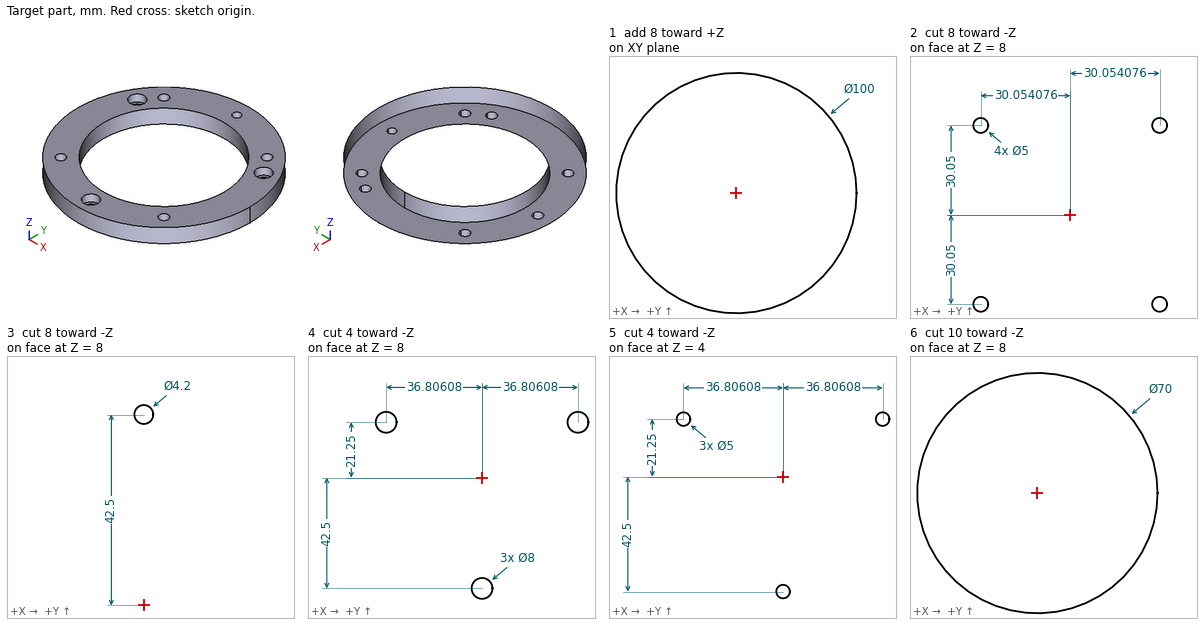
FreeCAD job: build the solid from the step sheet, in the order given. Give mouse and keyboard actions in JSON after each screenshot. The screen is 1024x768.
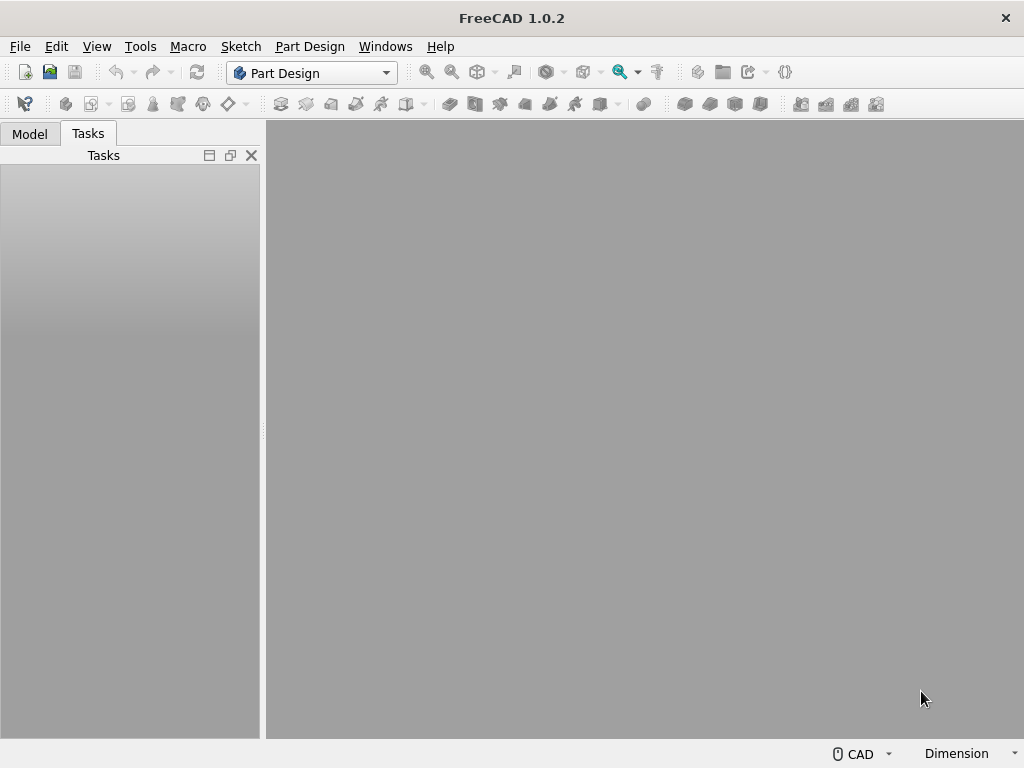
{"action": "left_click", "coordinate": [25, 72]}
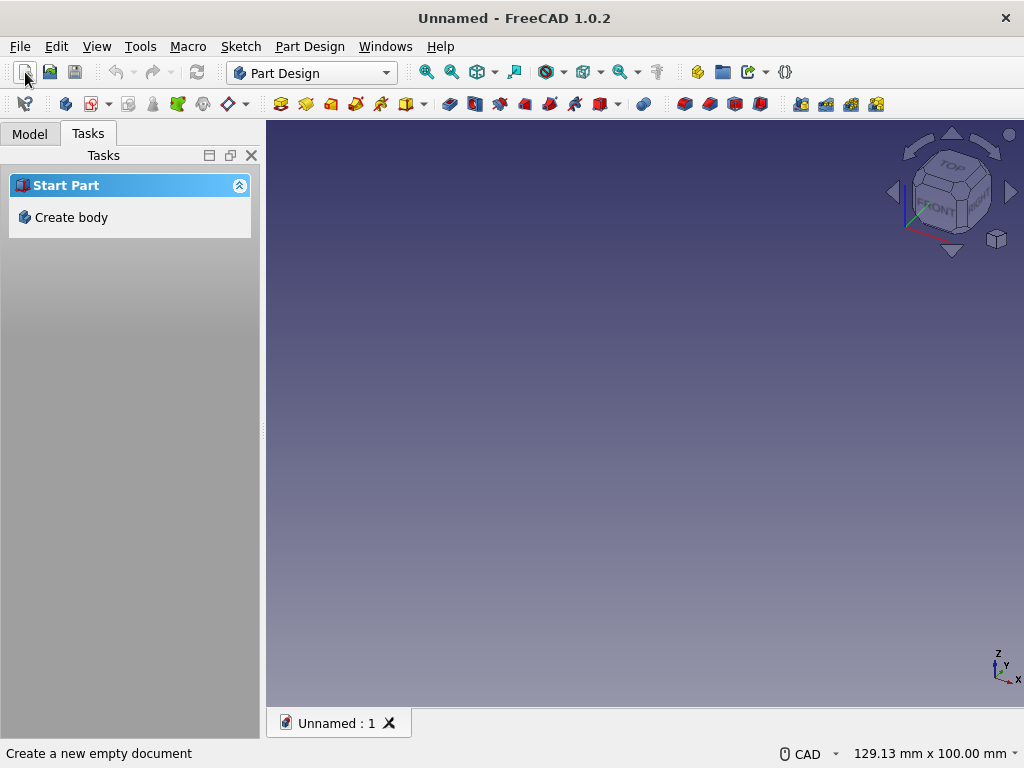
{"action": "left_click", "coordinate": [90, 104]}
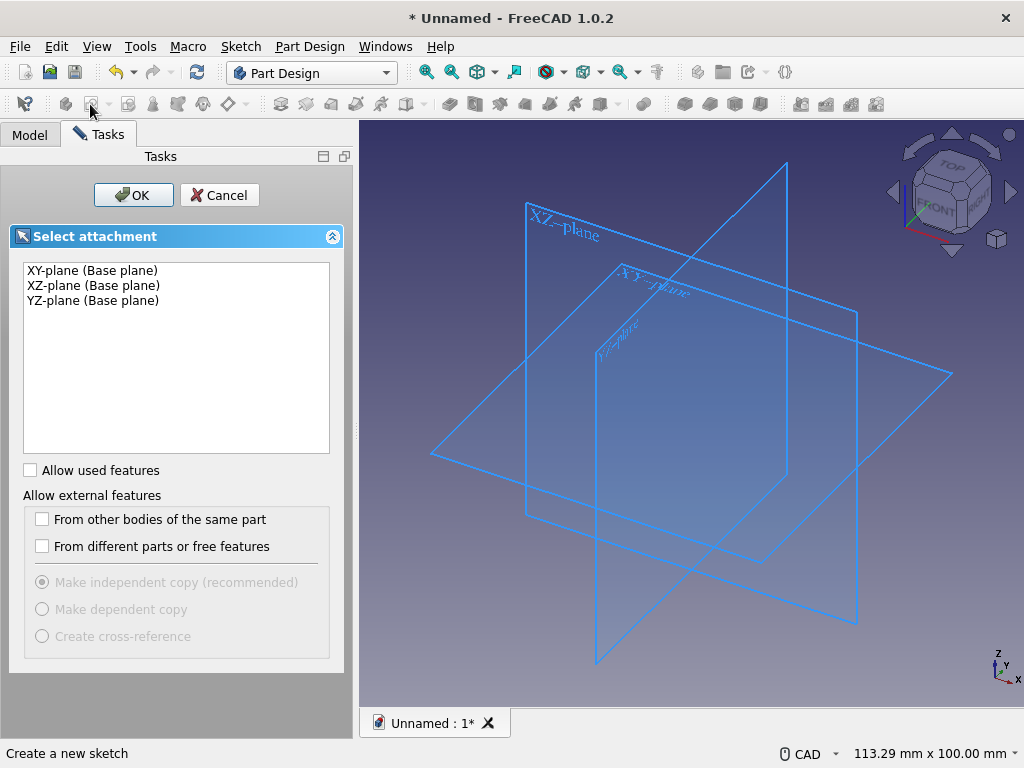
{"action": "left_click", "coordinate": [84, 270]}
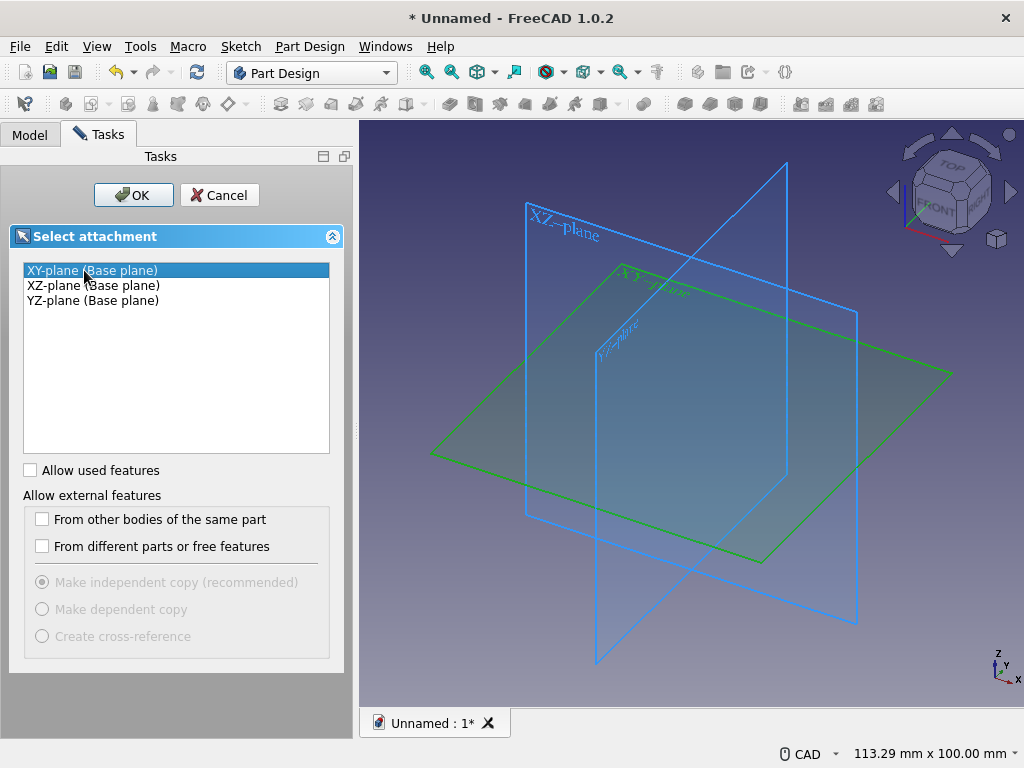
{"action": "left_click", "coordinate": [134, 195]}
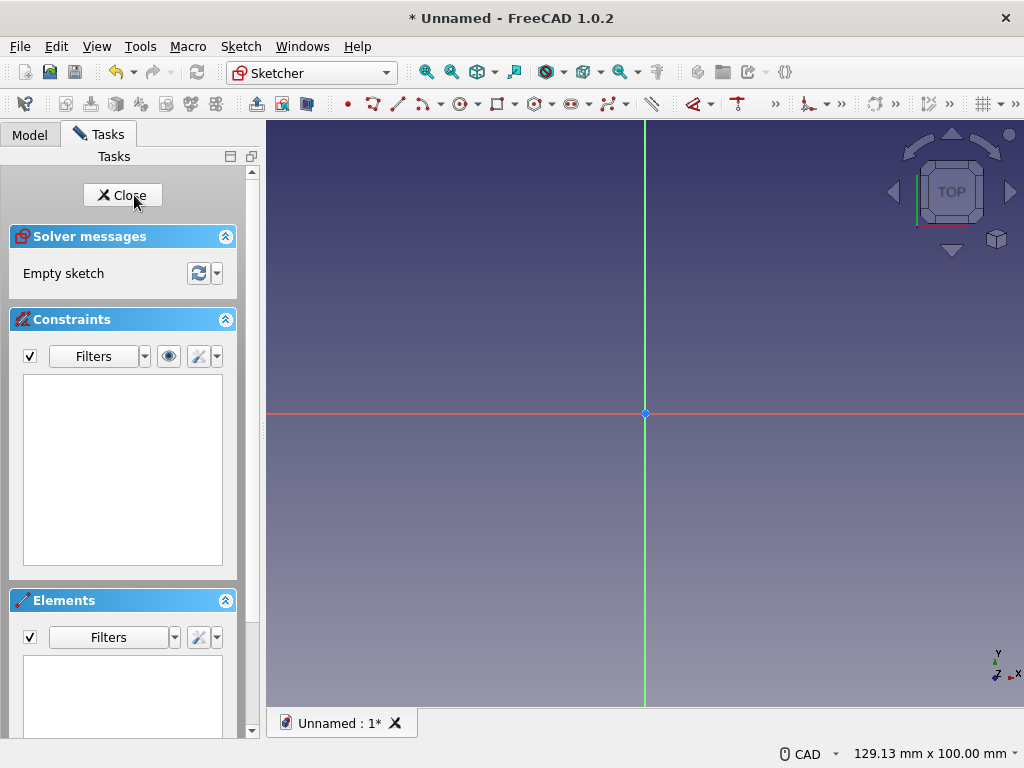
{"action": "scroll", "coordinate": [437, 414], "scroll_direction": "down", "scroll_amount": 2}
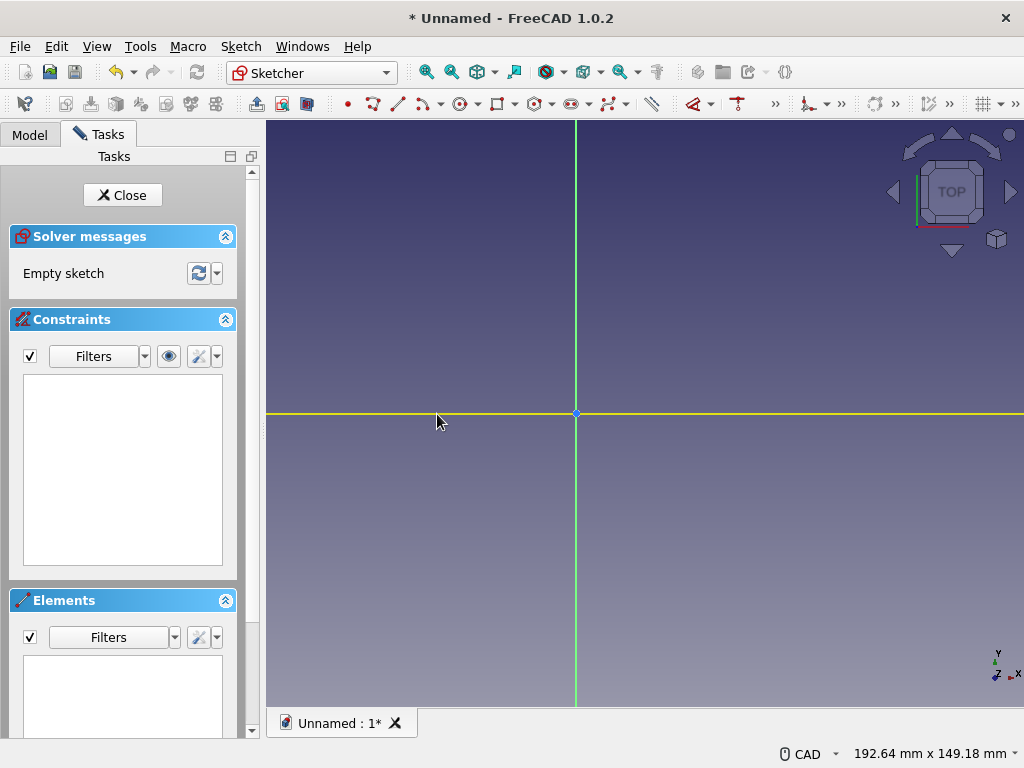
{"action": "key", "text": "g c"}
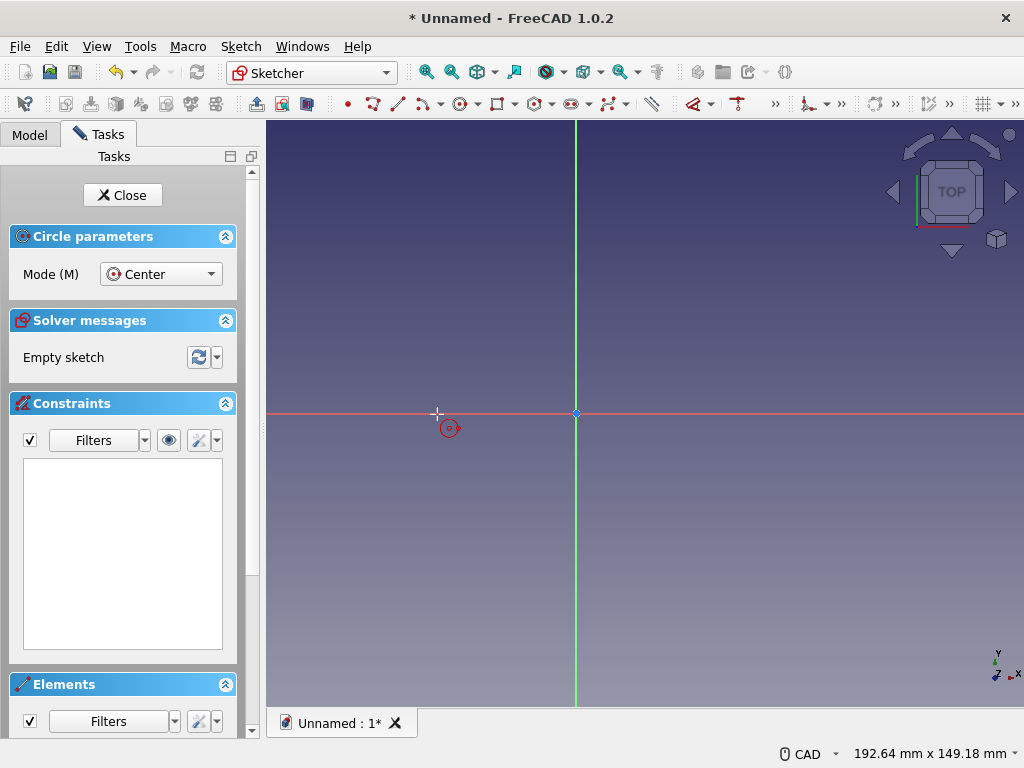
{"action": "left_click", "coordinate": [577, 414]}
{"action": "mouse_move", "coordinate": [716, 275]}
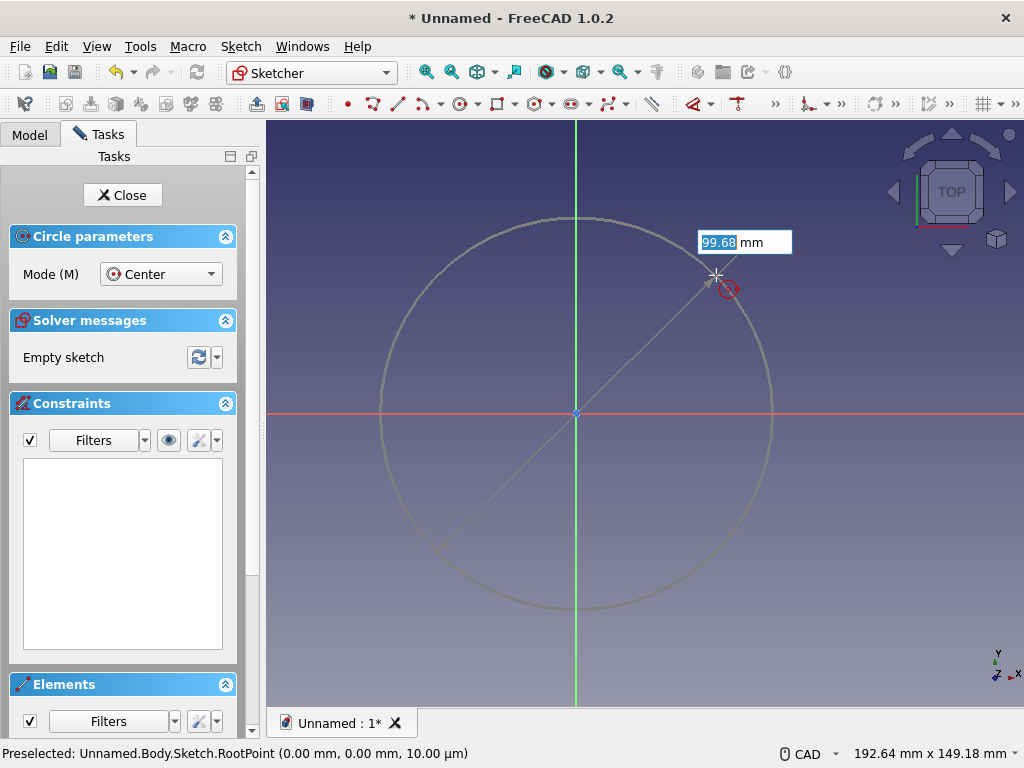
{"action": "type", "text": "100"}
{"action": "key", "text": "Return"}
{"action": "key", "text": "Escape"}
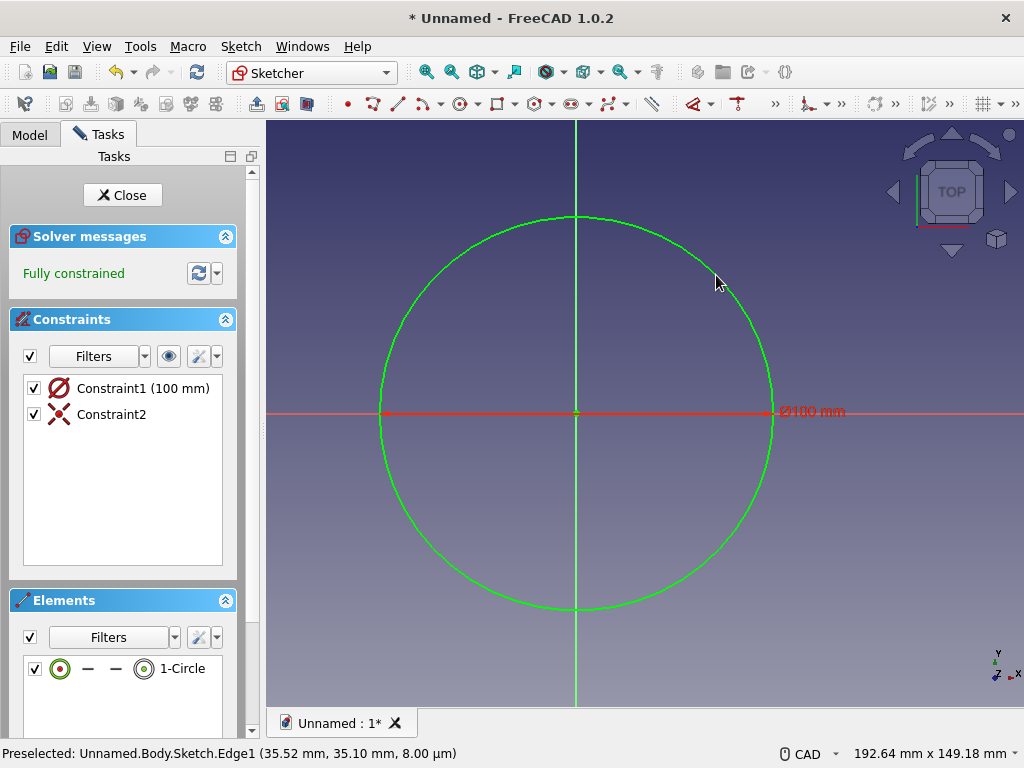
{"action": "left_click", "coordinate": [123, 195]}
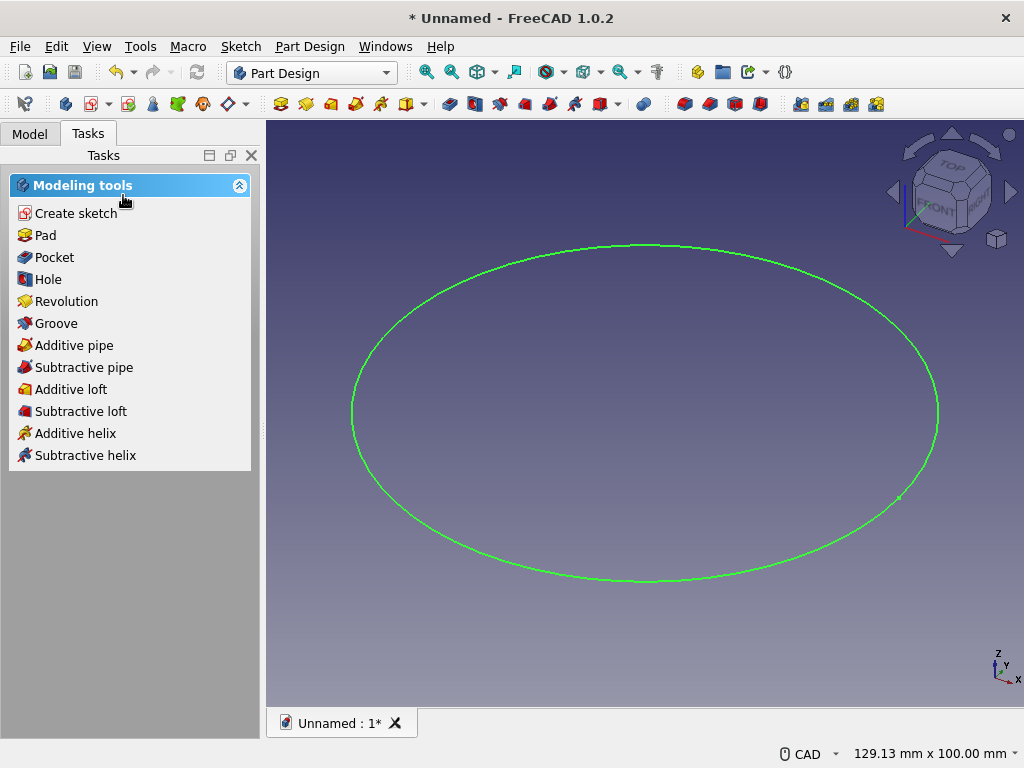
{"action": "left_click", "coordinate": [281, 104]}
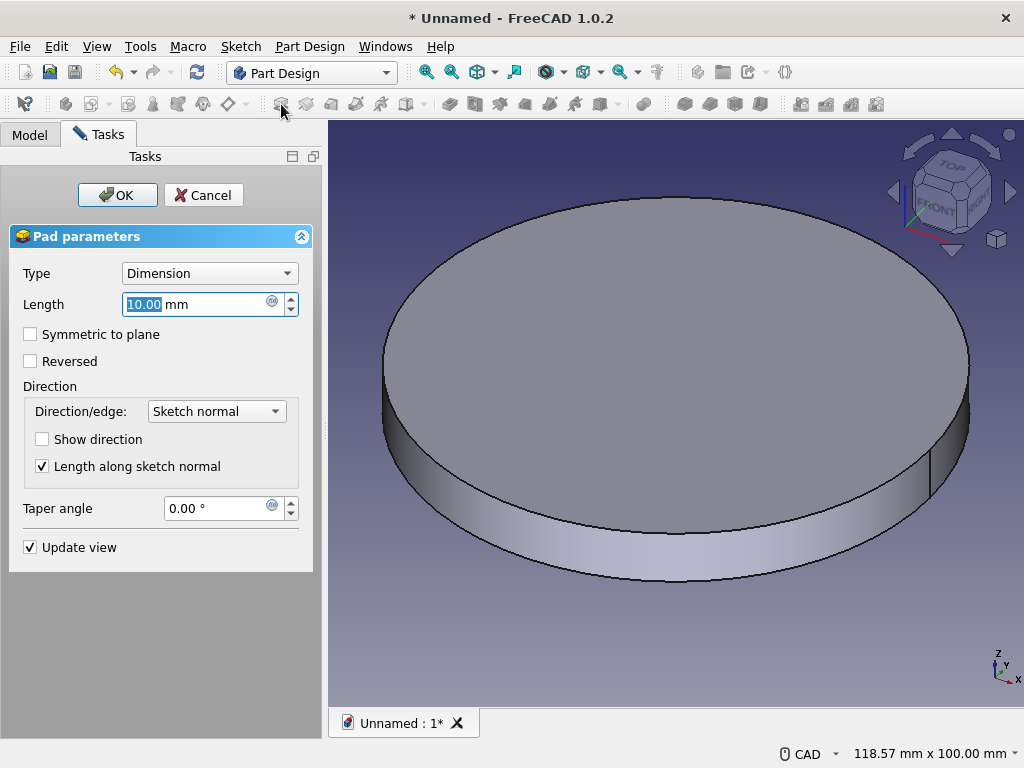
{"action": "type", "text": "8"}
{"action": "key", "text": "Tab"}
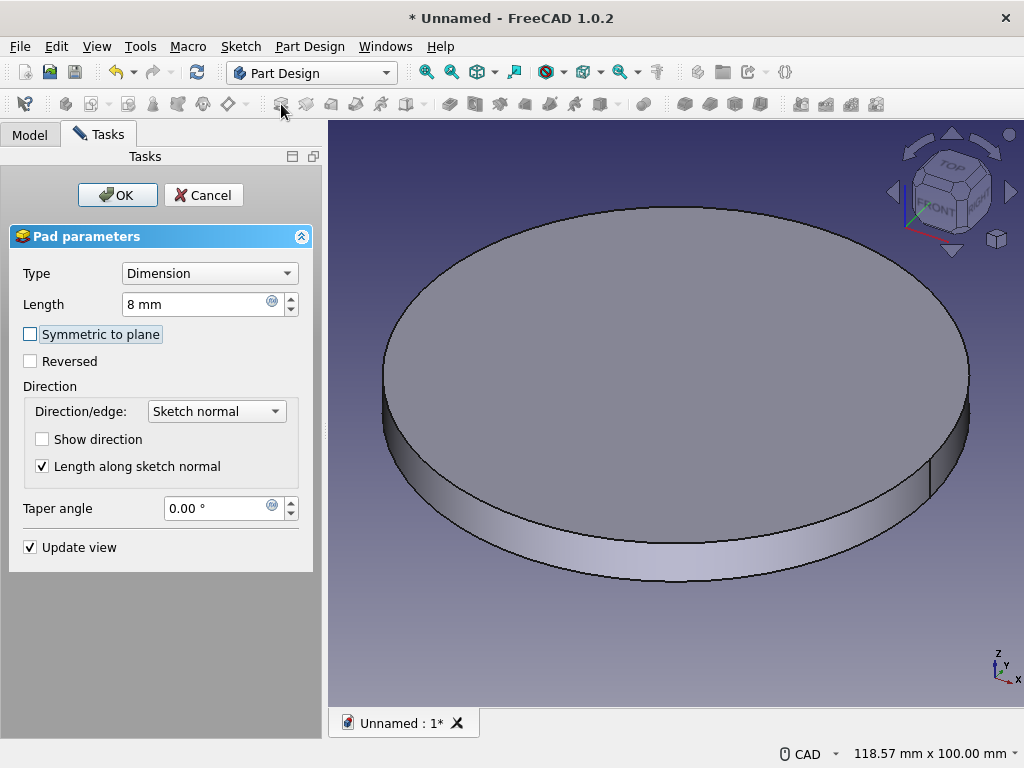
{"action": "left_click", "coordinate": [118, 195]}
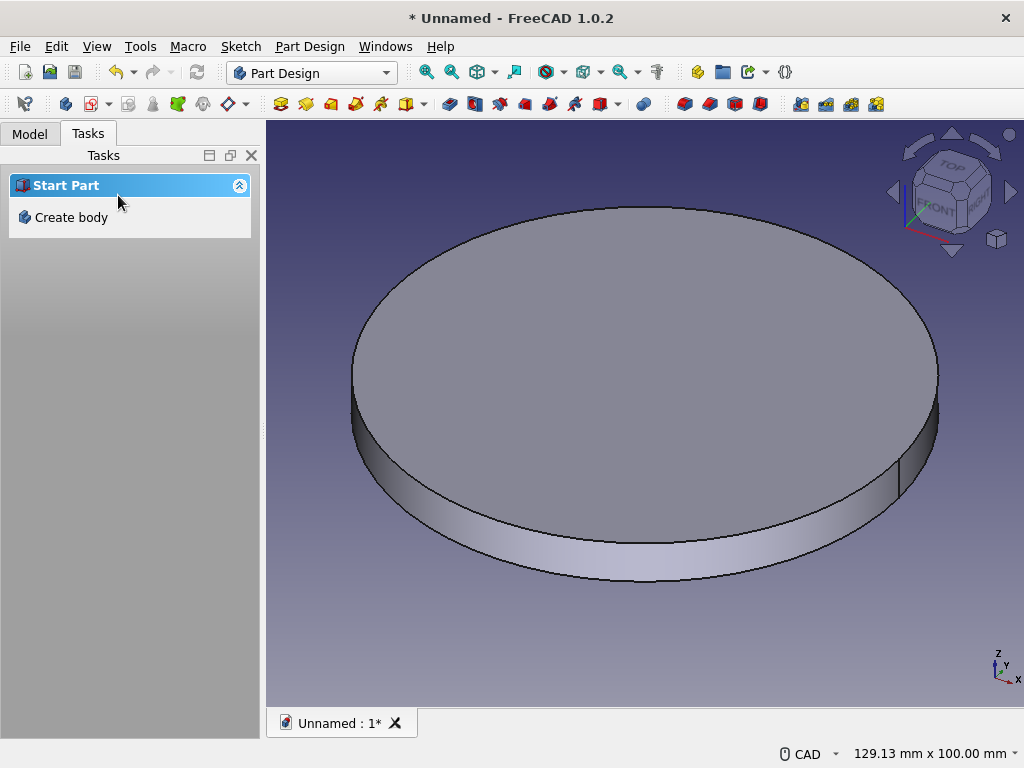
{"action": "left_click", "coordinate": [427, 72]}